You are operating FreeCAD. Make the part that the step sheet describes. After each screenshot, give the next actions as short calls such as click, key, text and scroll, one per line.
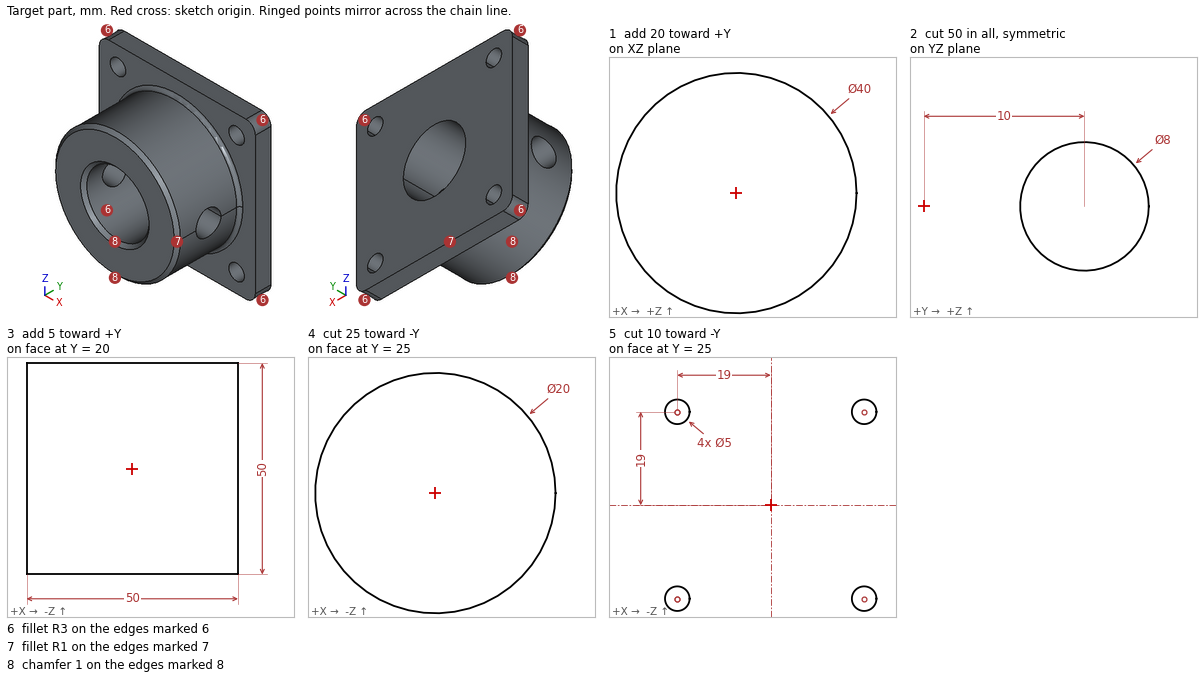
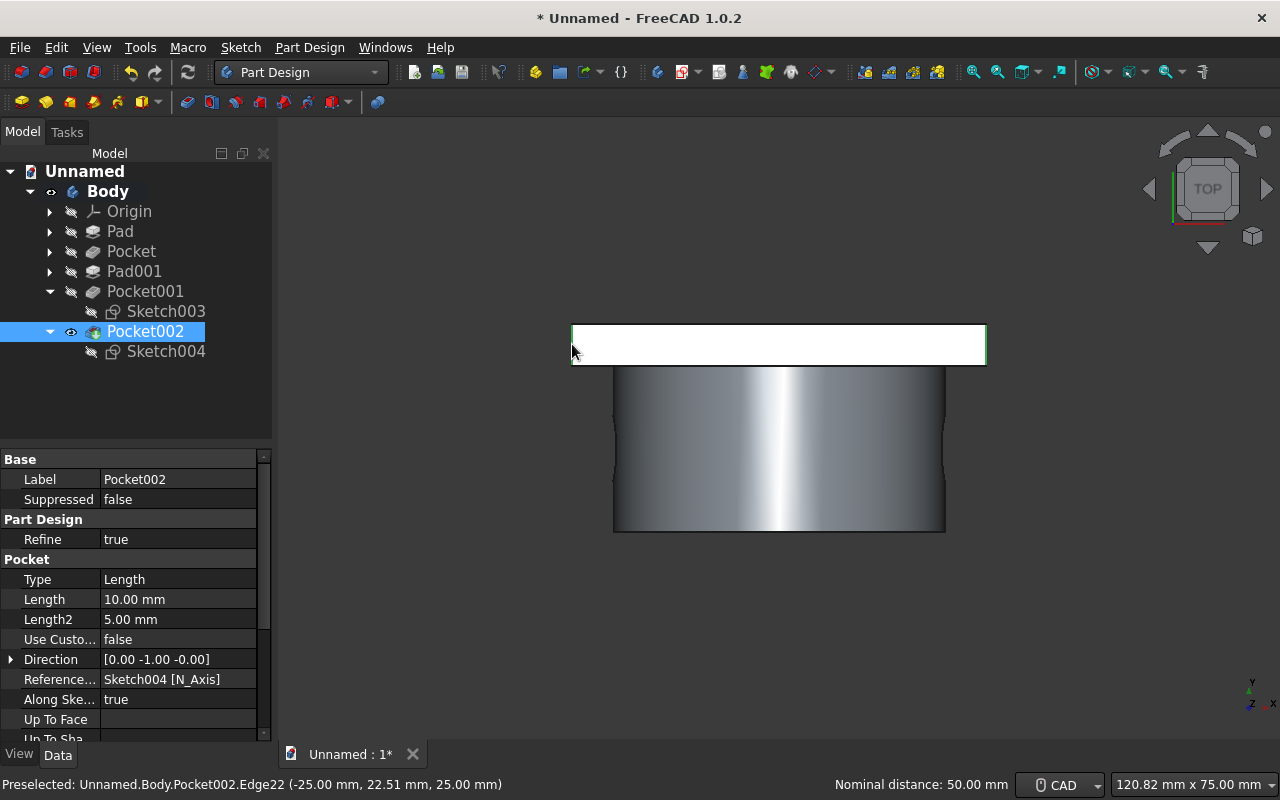
key(1)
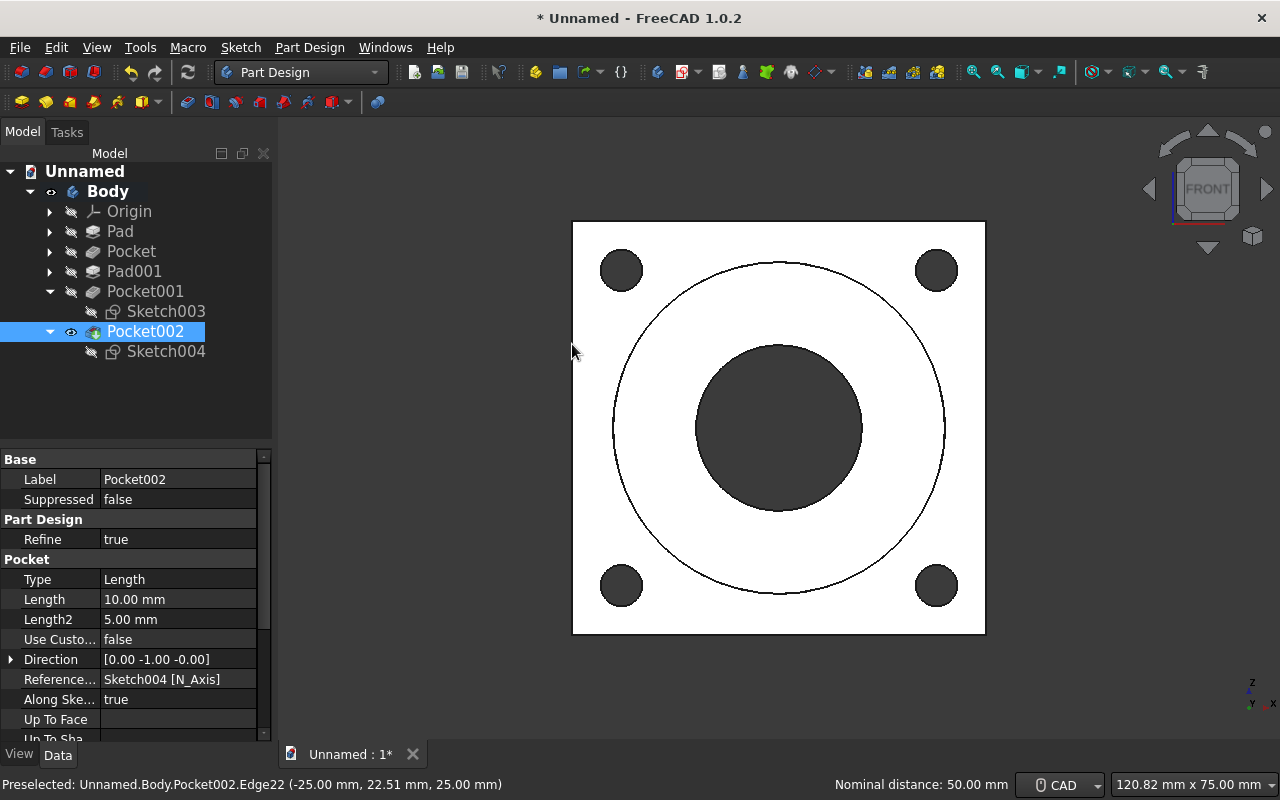
key(3)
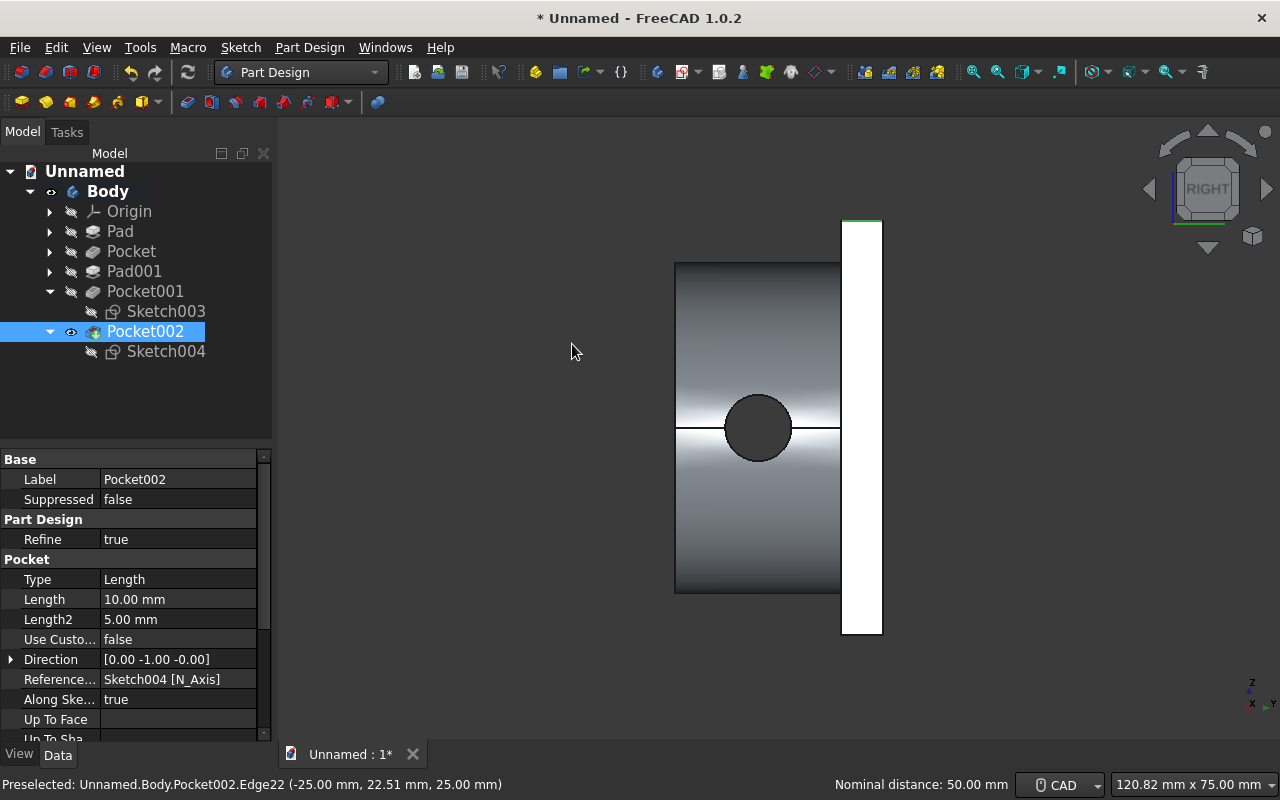
click(862, 634, ctrl)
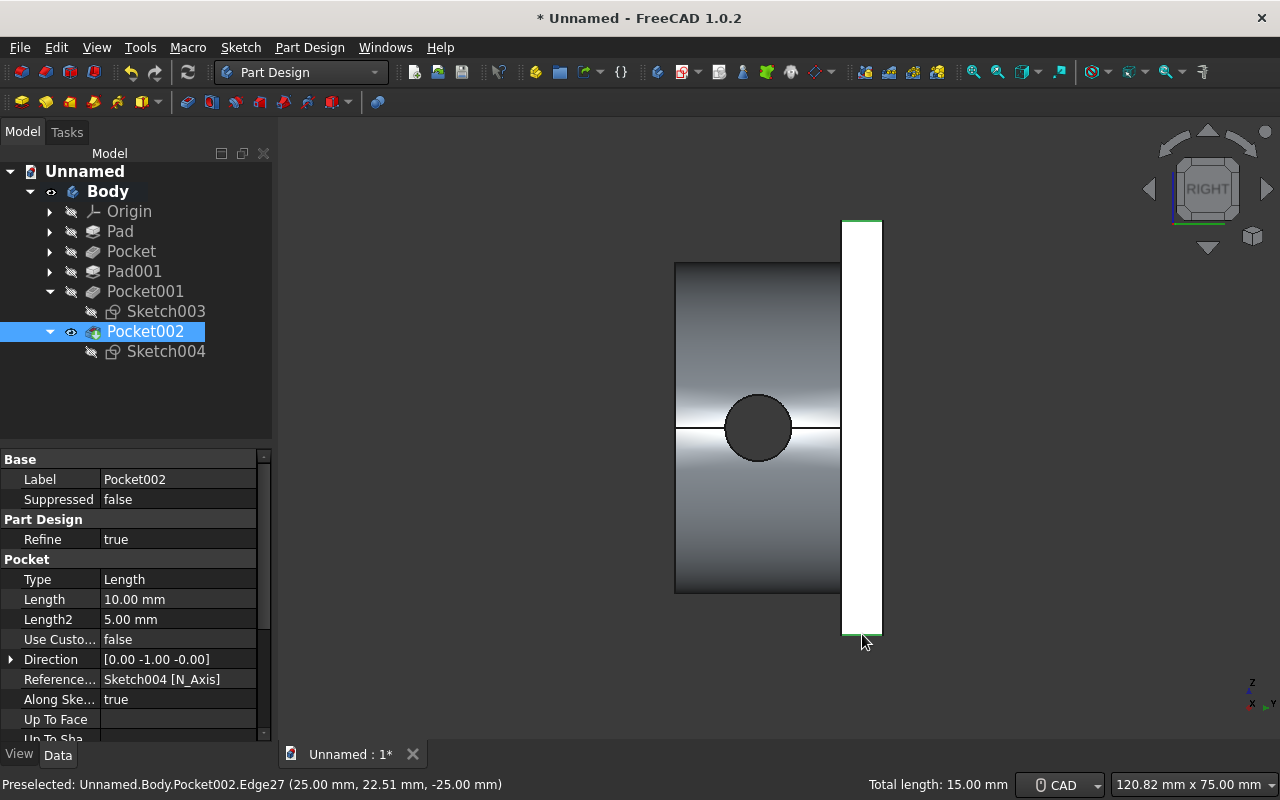
key(5)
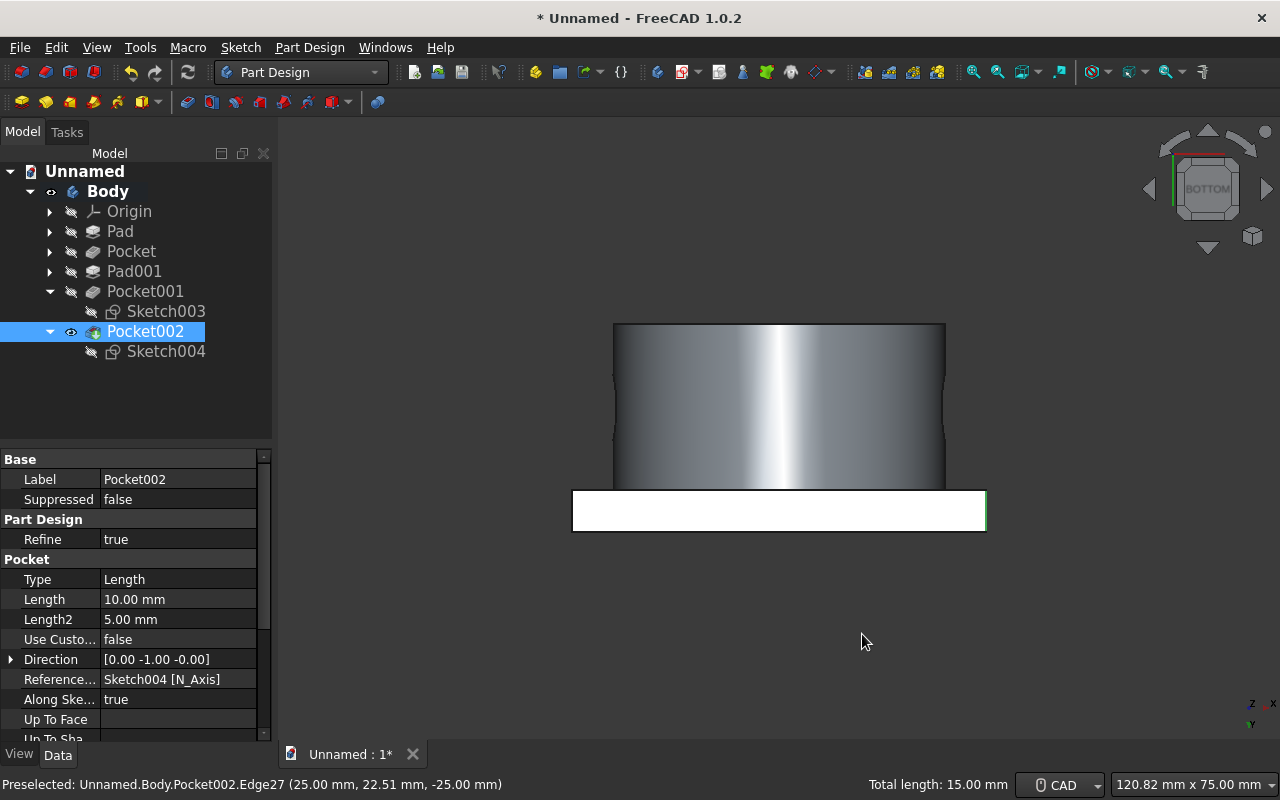
click(974, 72)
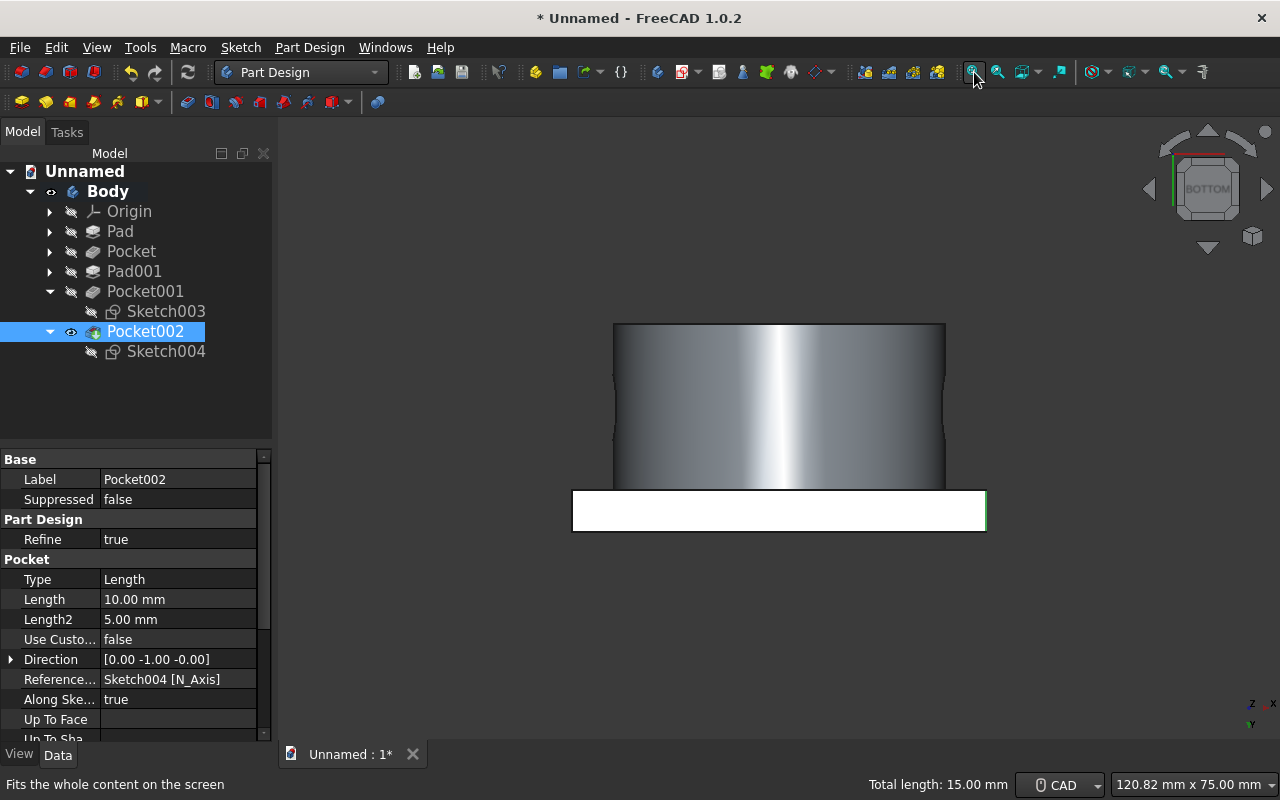
click(572, 510, ctrl)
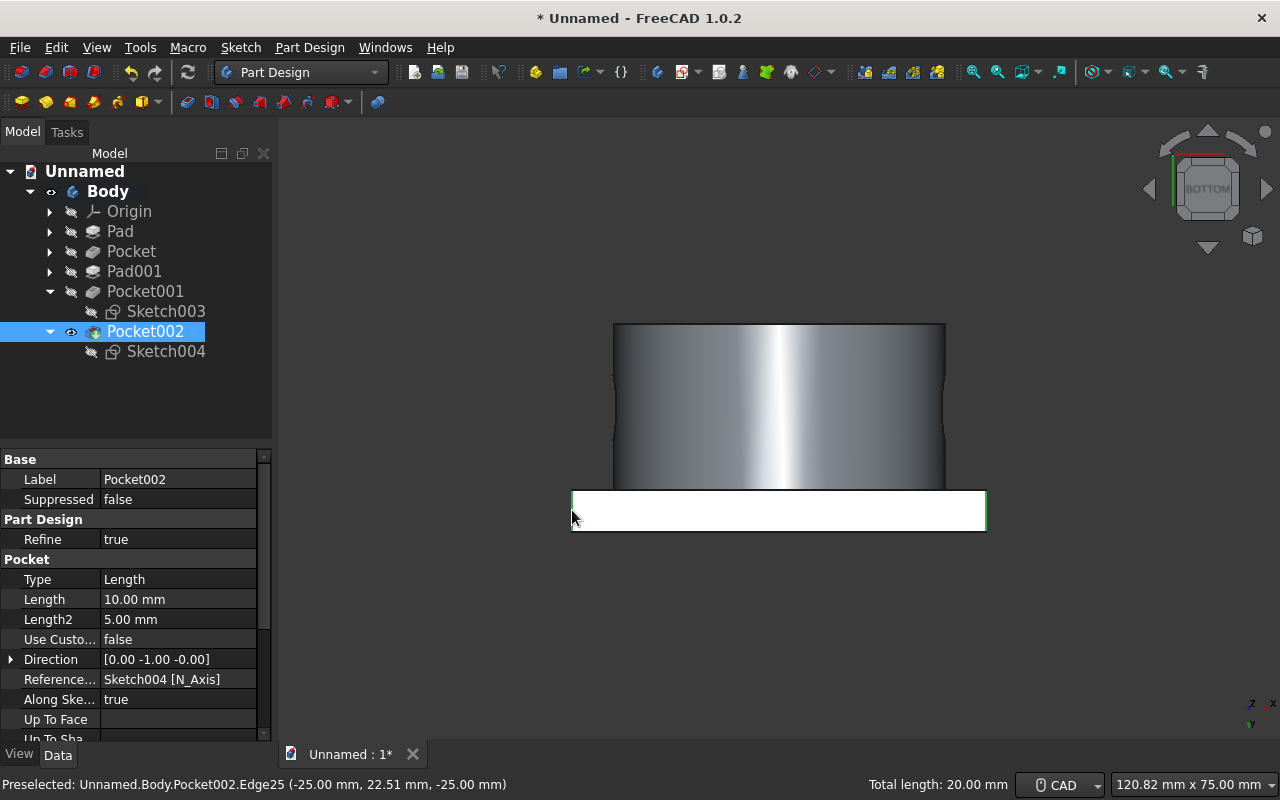
click(22, 72)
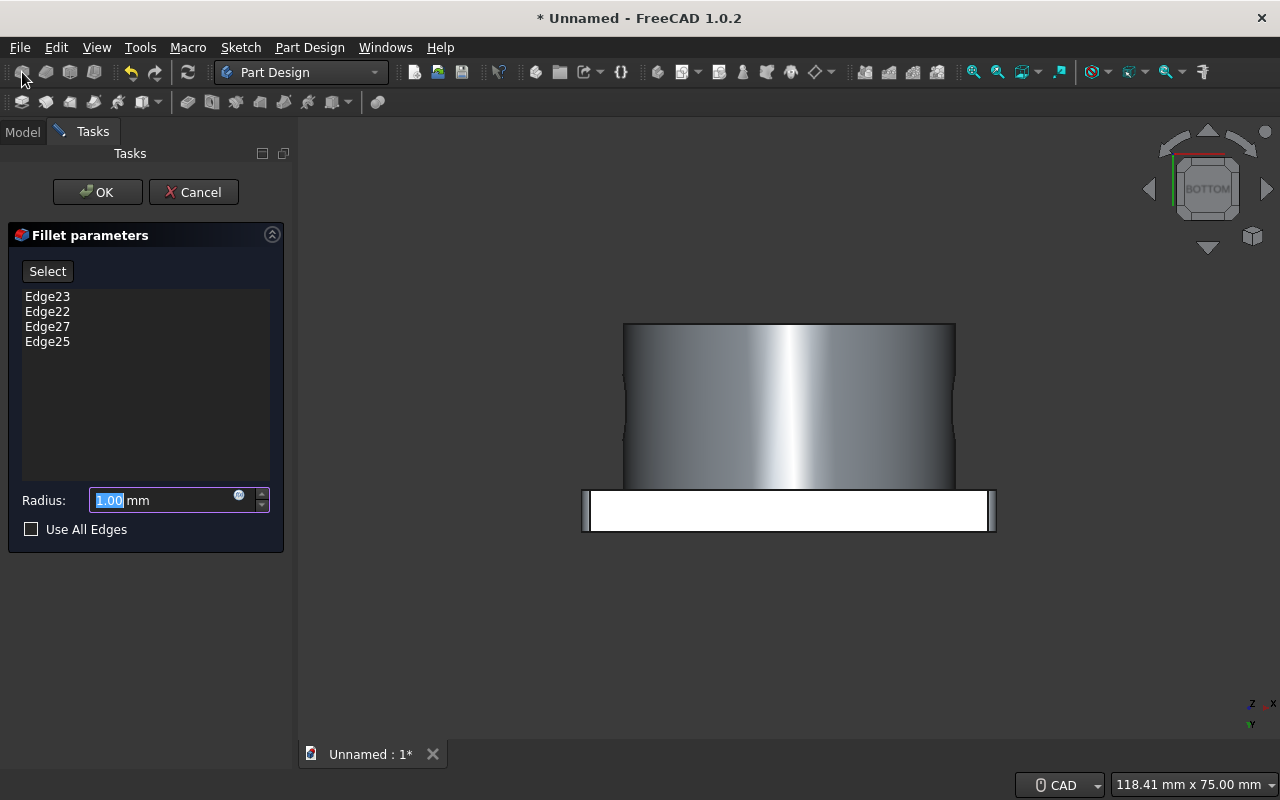
text(3)
key(Tab)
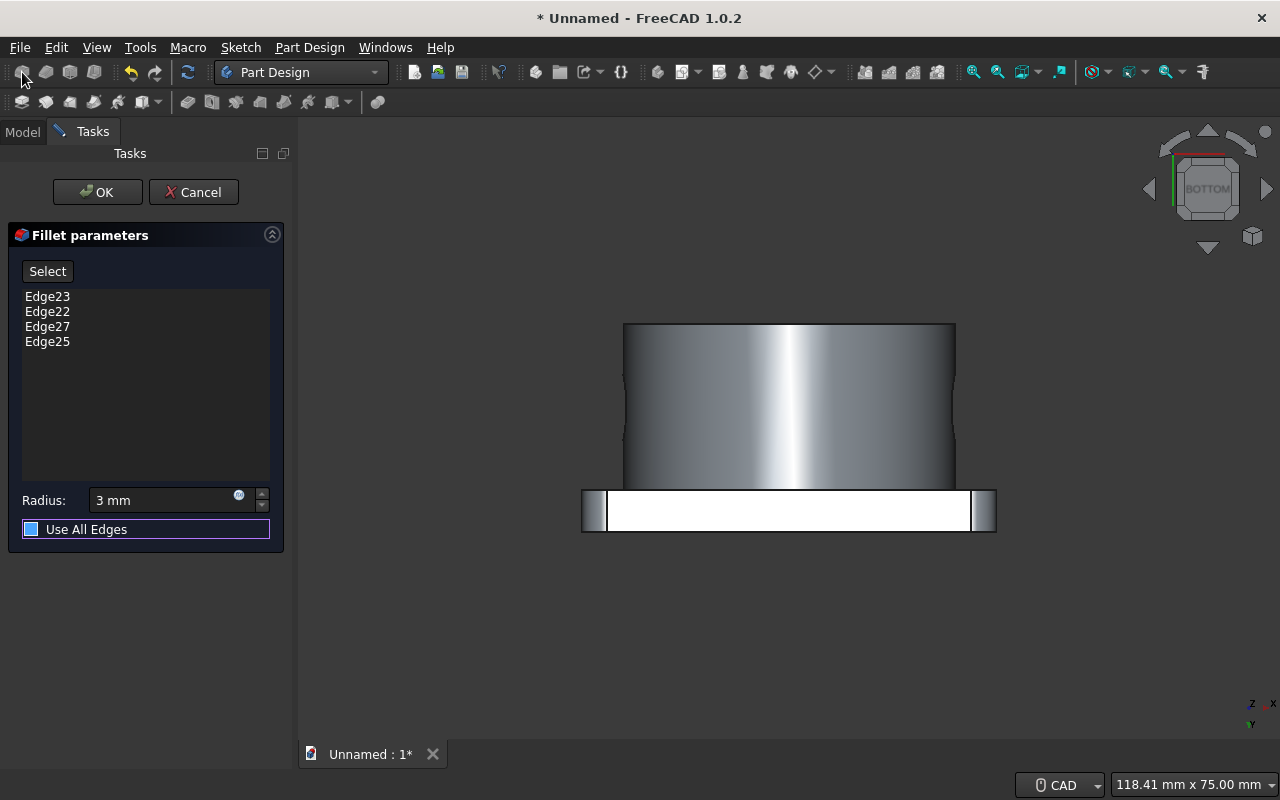
click(98, 192)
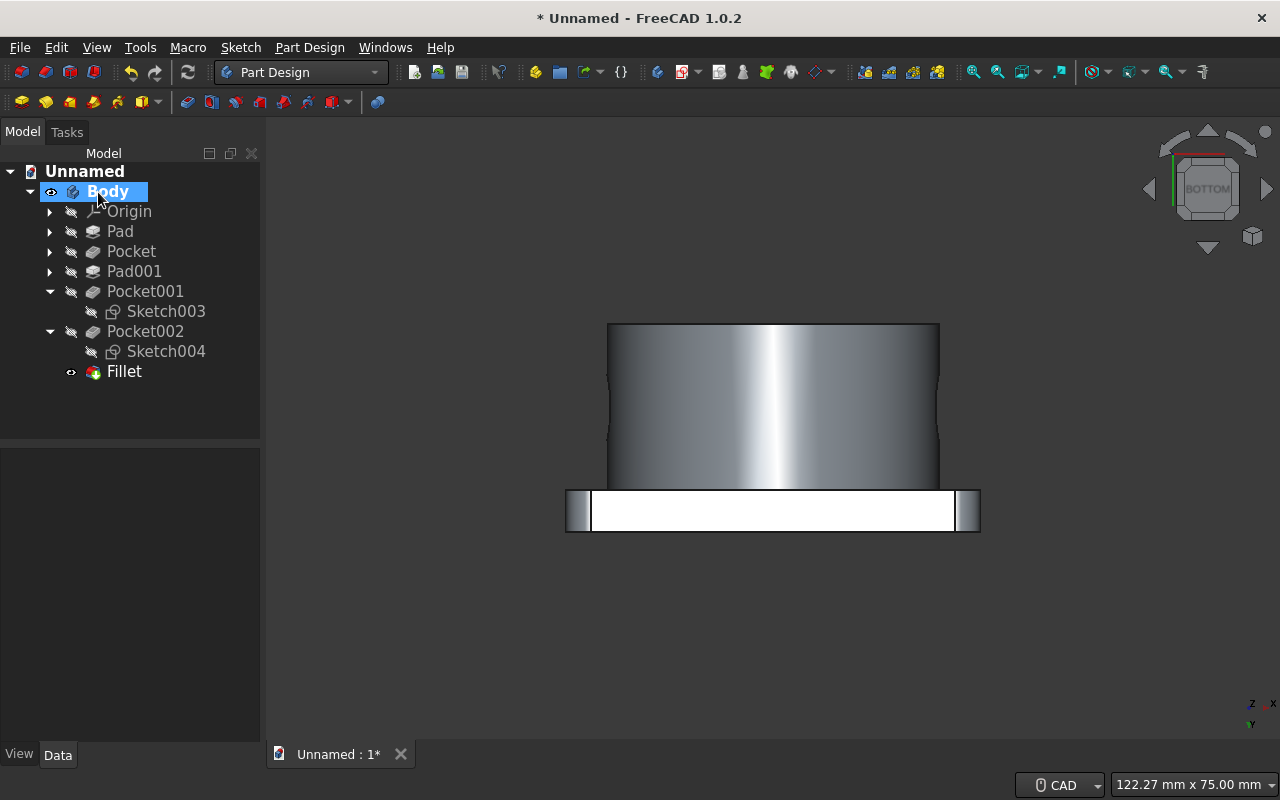
key(v)
key(f)